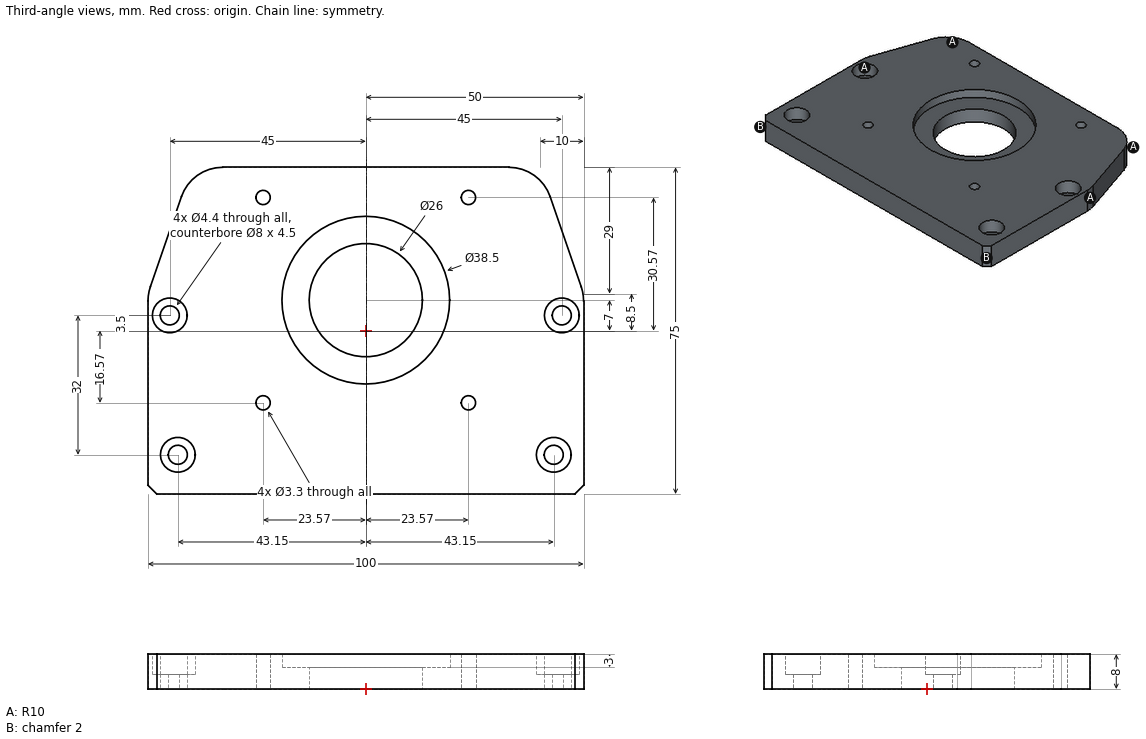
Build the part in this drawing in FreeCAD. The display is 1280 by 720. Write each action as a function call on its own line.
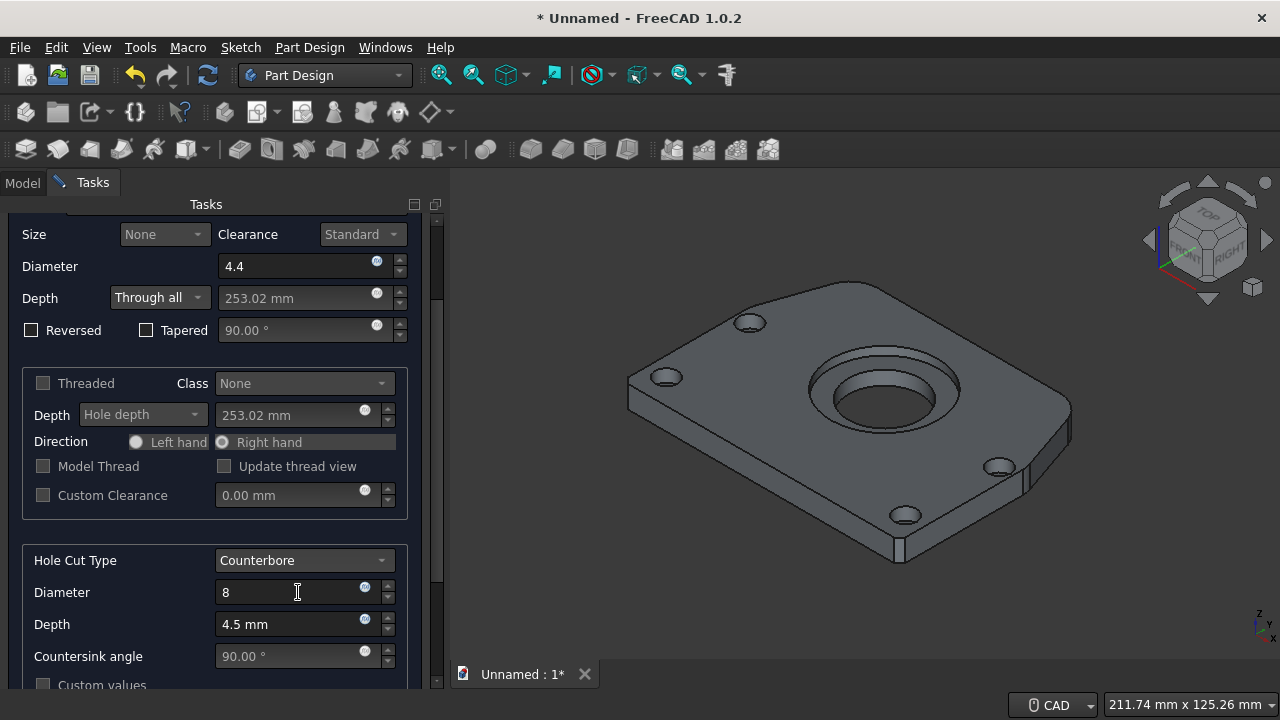
scroll(437, 451, up, 3)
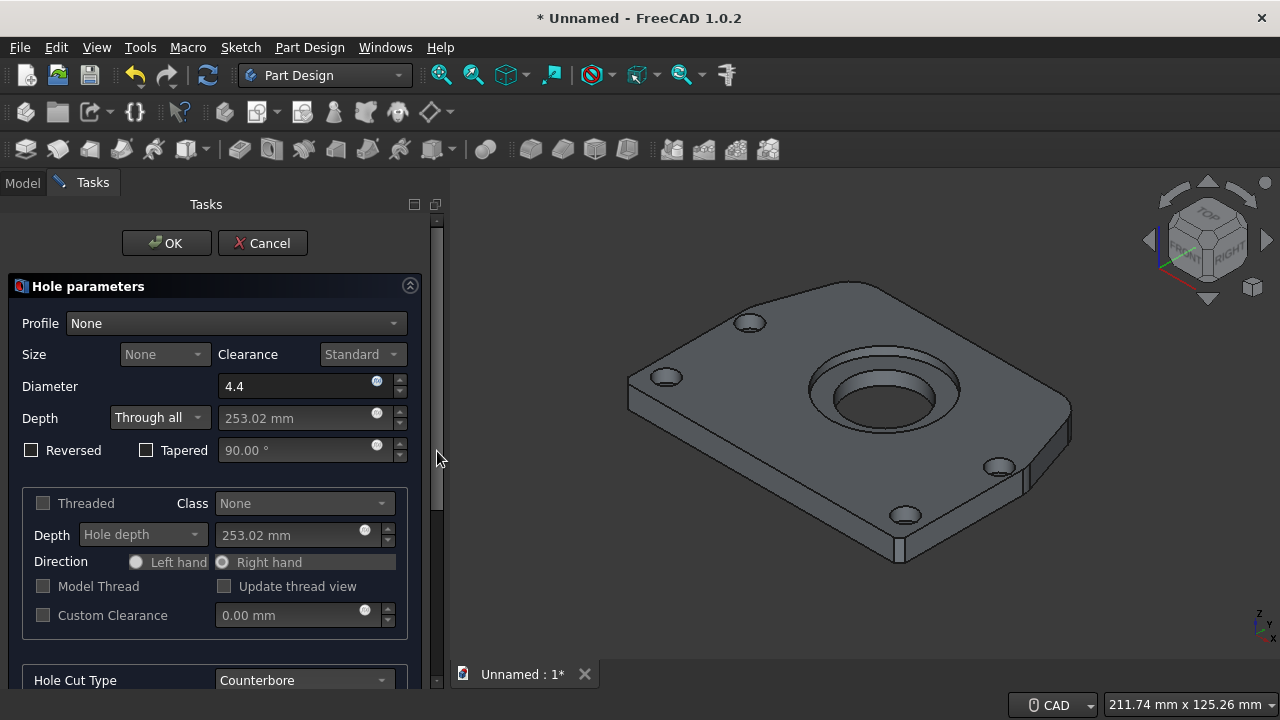
click(167, 243)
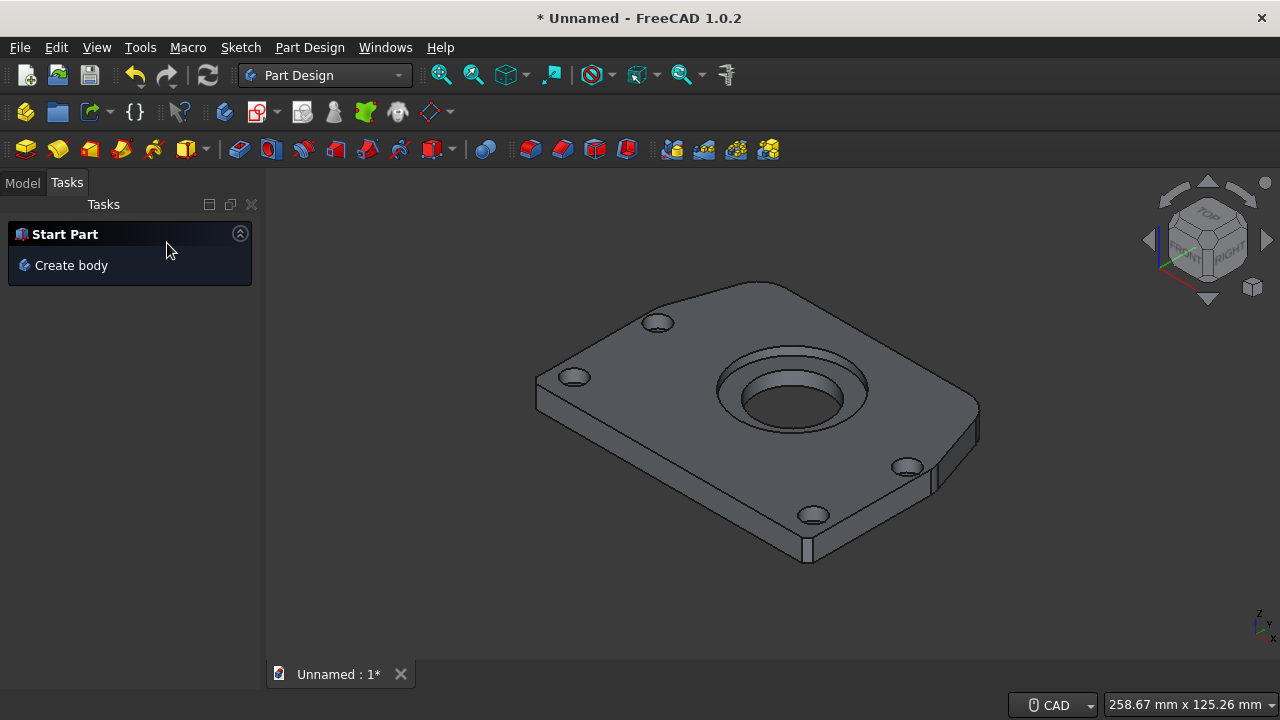
click(822, 463)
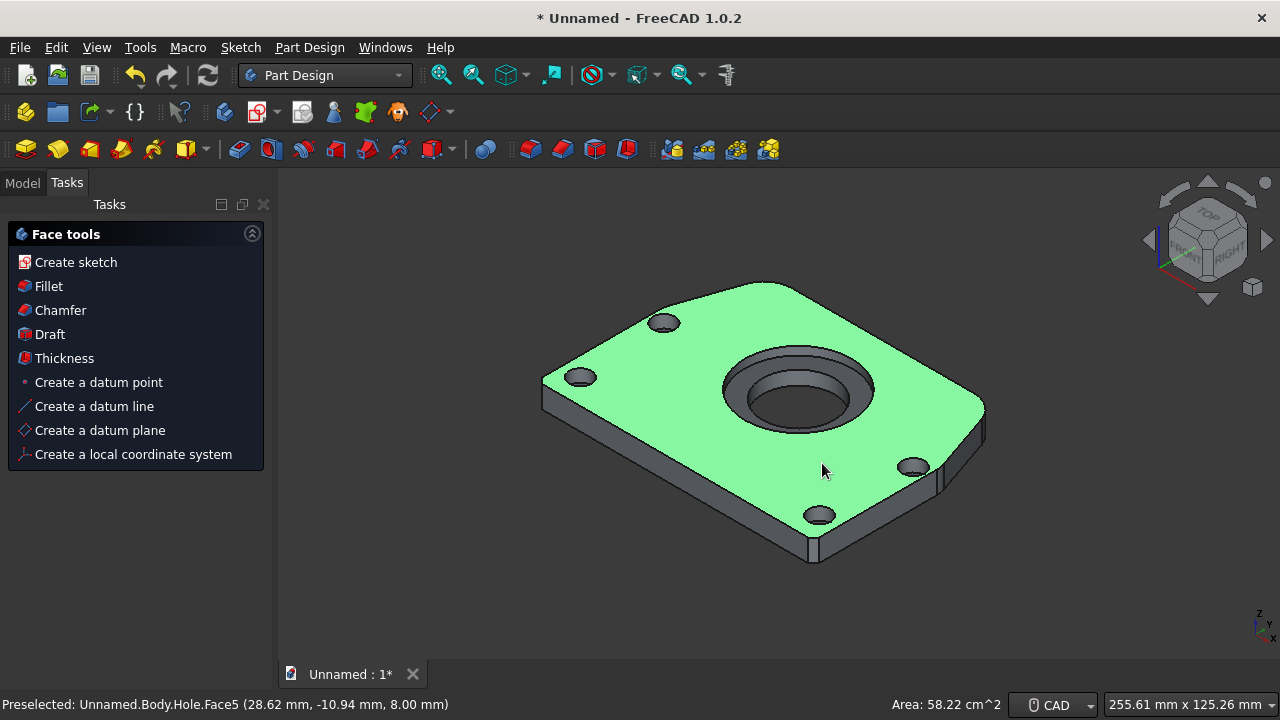
click(258, 112)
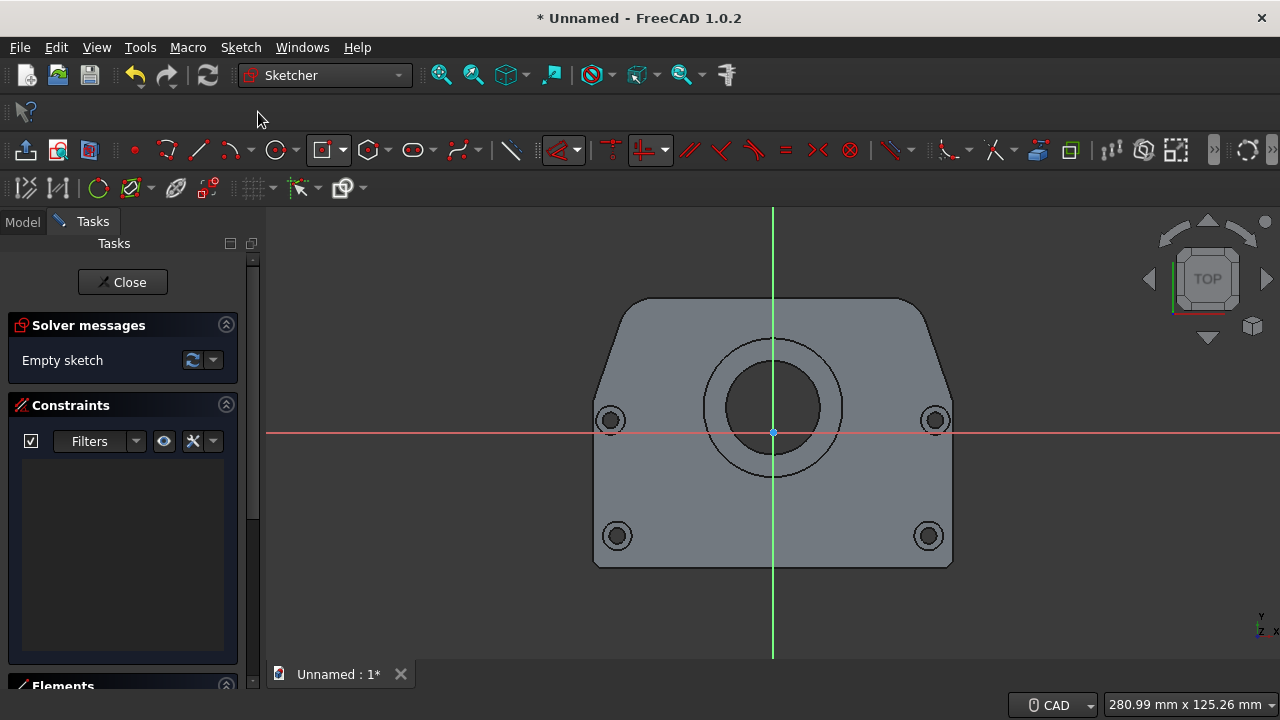
scroll(912, 356, up, 2)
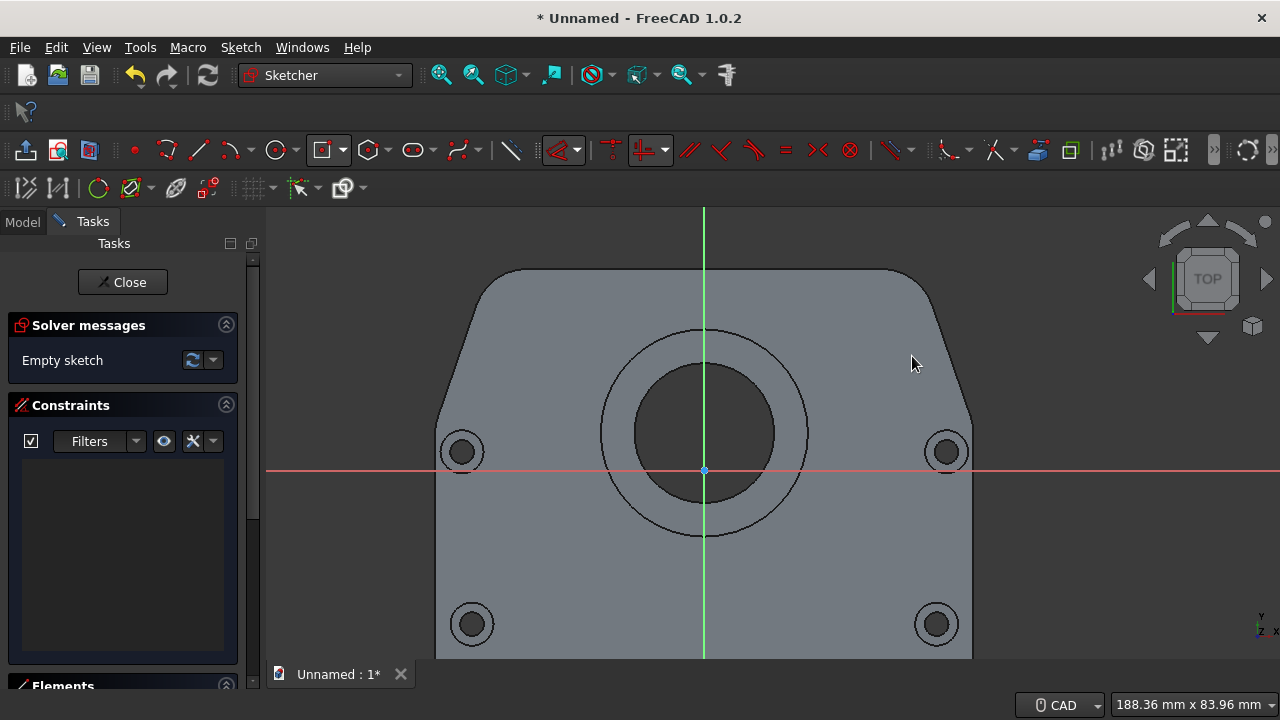
click(276, 150)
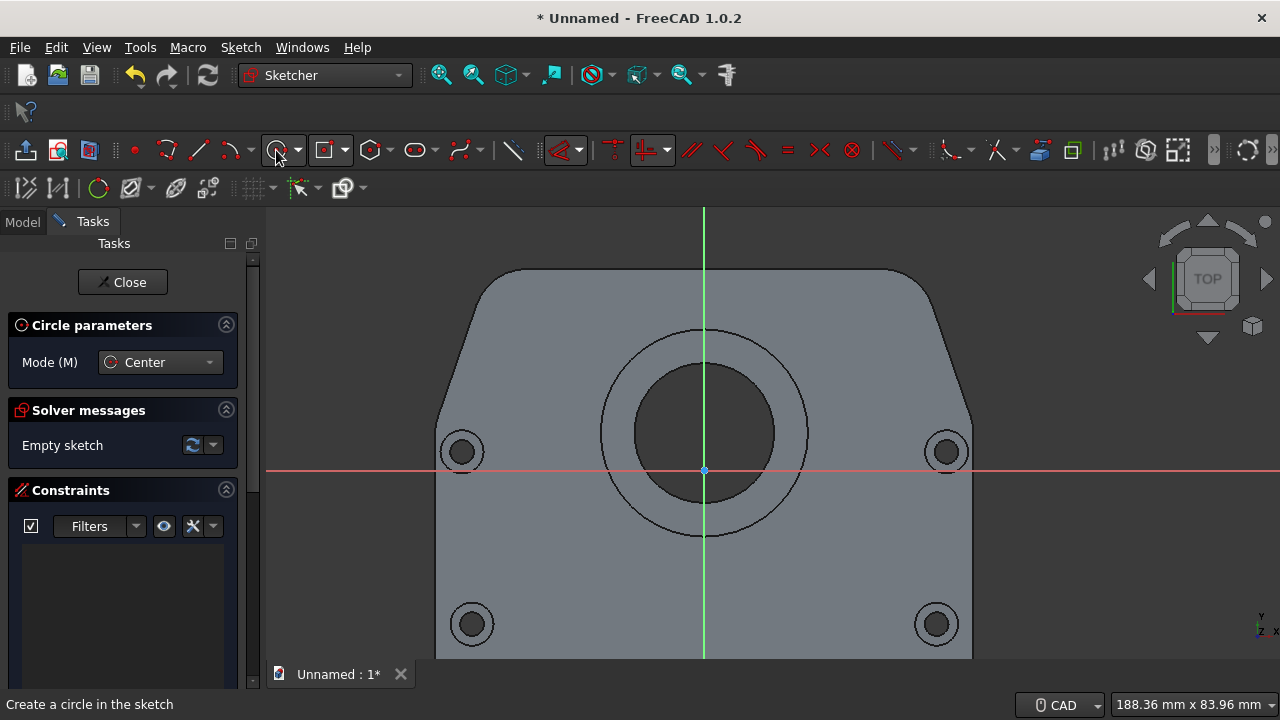
scroll(577, 560, up, 5)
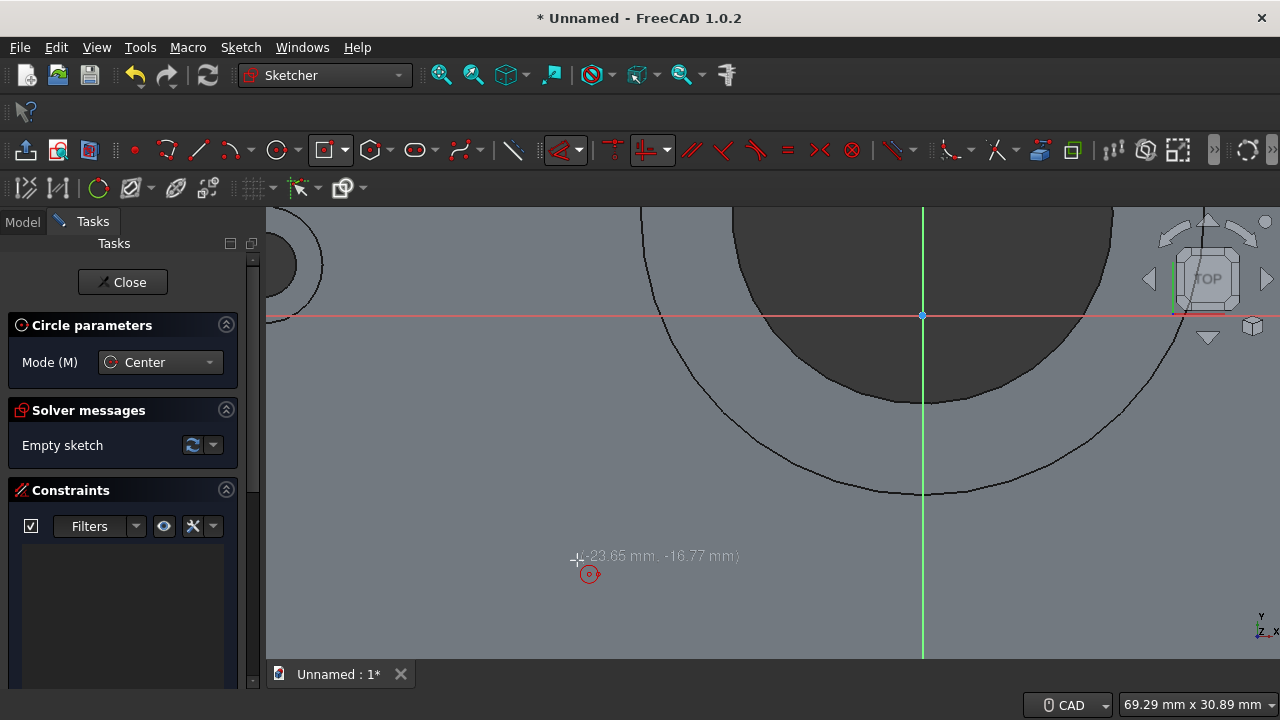
click(578, 558)
click(595, 541)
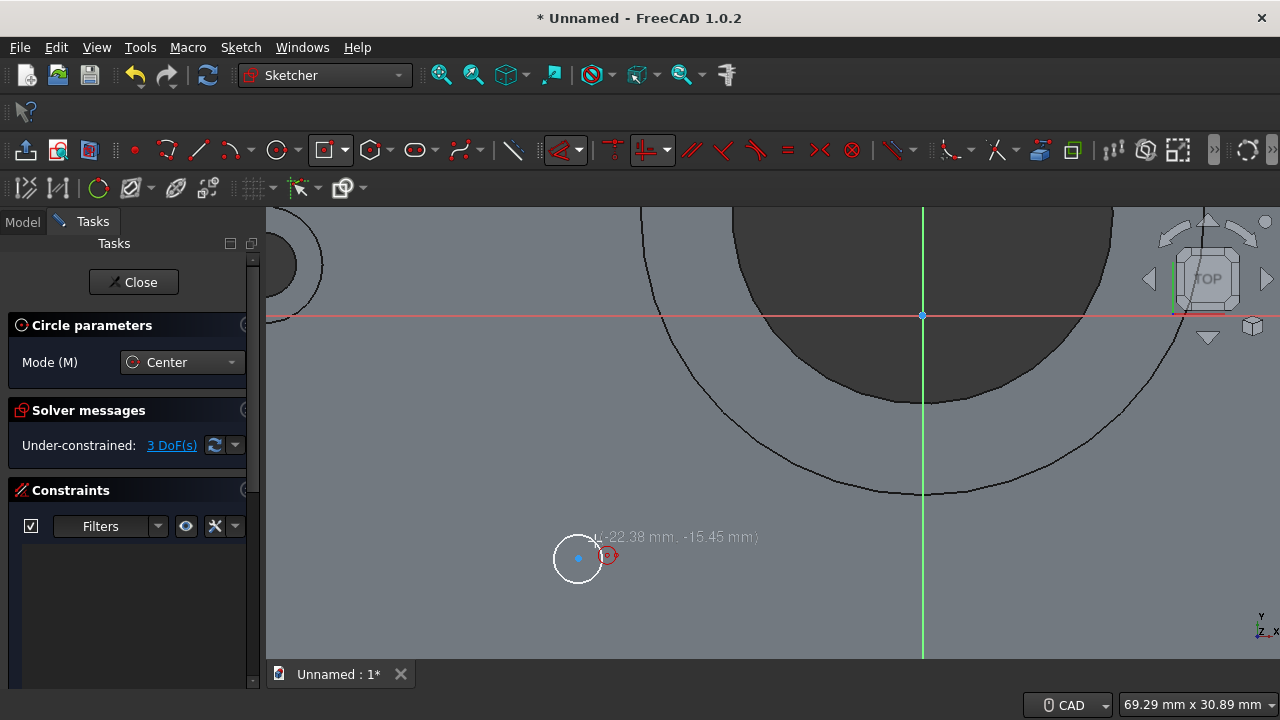
scroll(578, 561, down, 5)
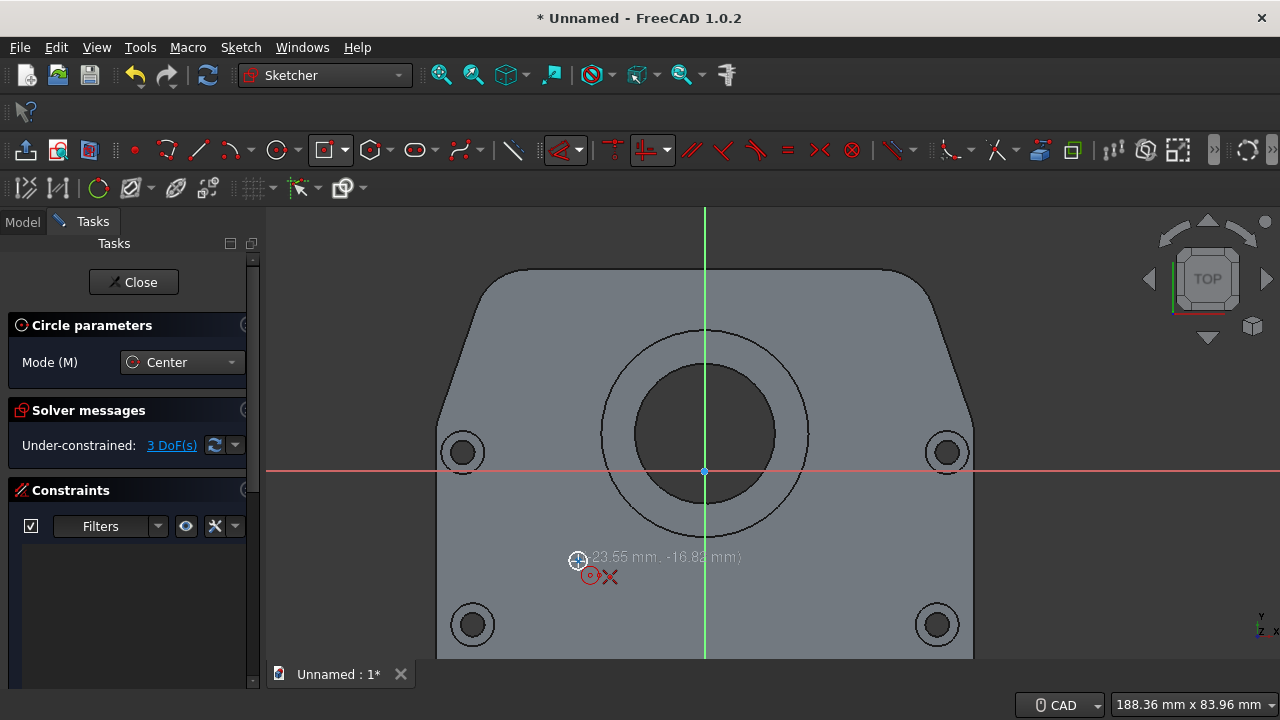
scroll(832, 561, up, 5)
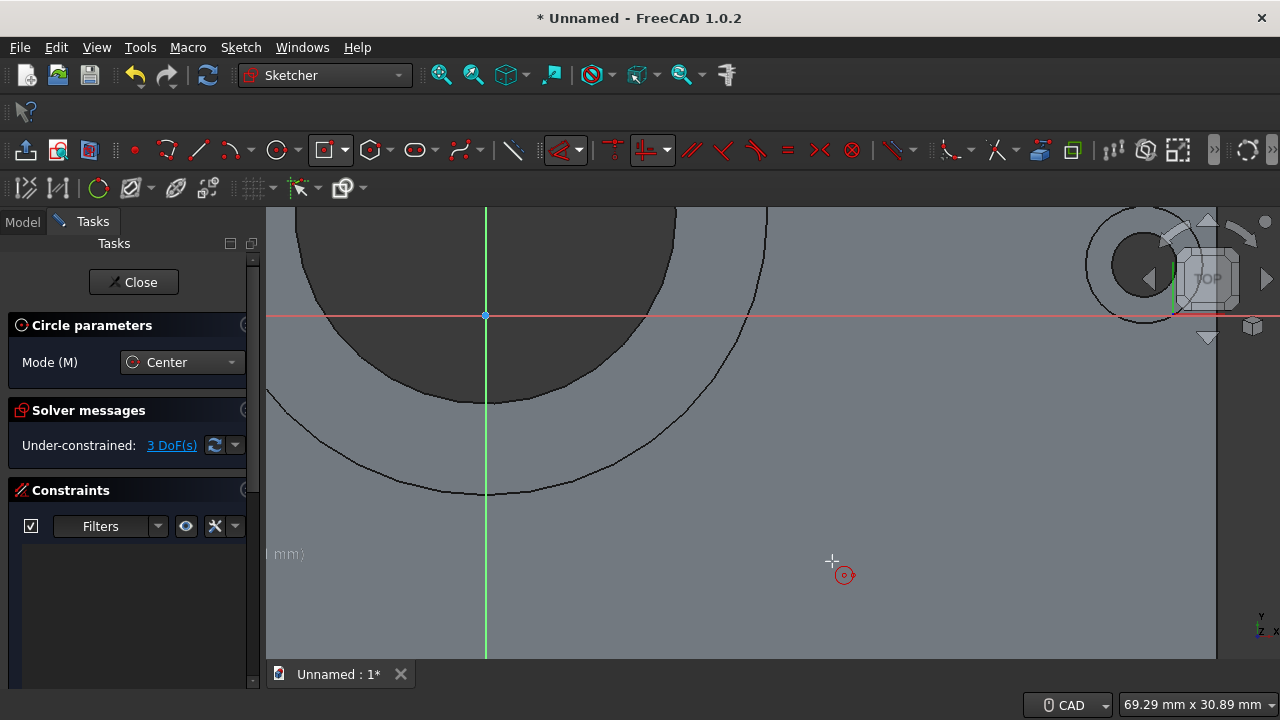
click(831, 558)
click(848, 541)